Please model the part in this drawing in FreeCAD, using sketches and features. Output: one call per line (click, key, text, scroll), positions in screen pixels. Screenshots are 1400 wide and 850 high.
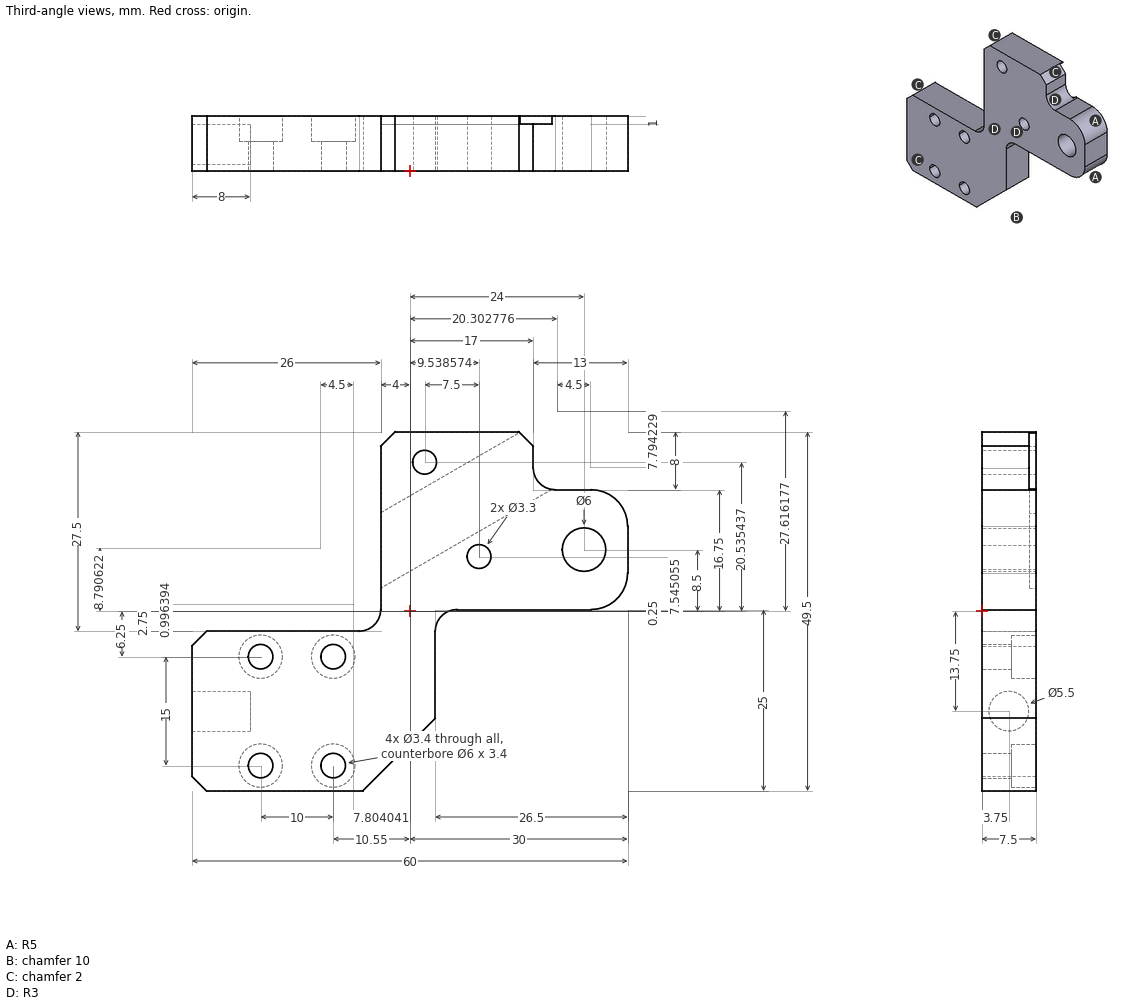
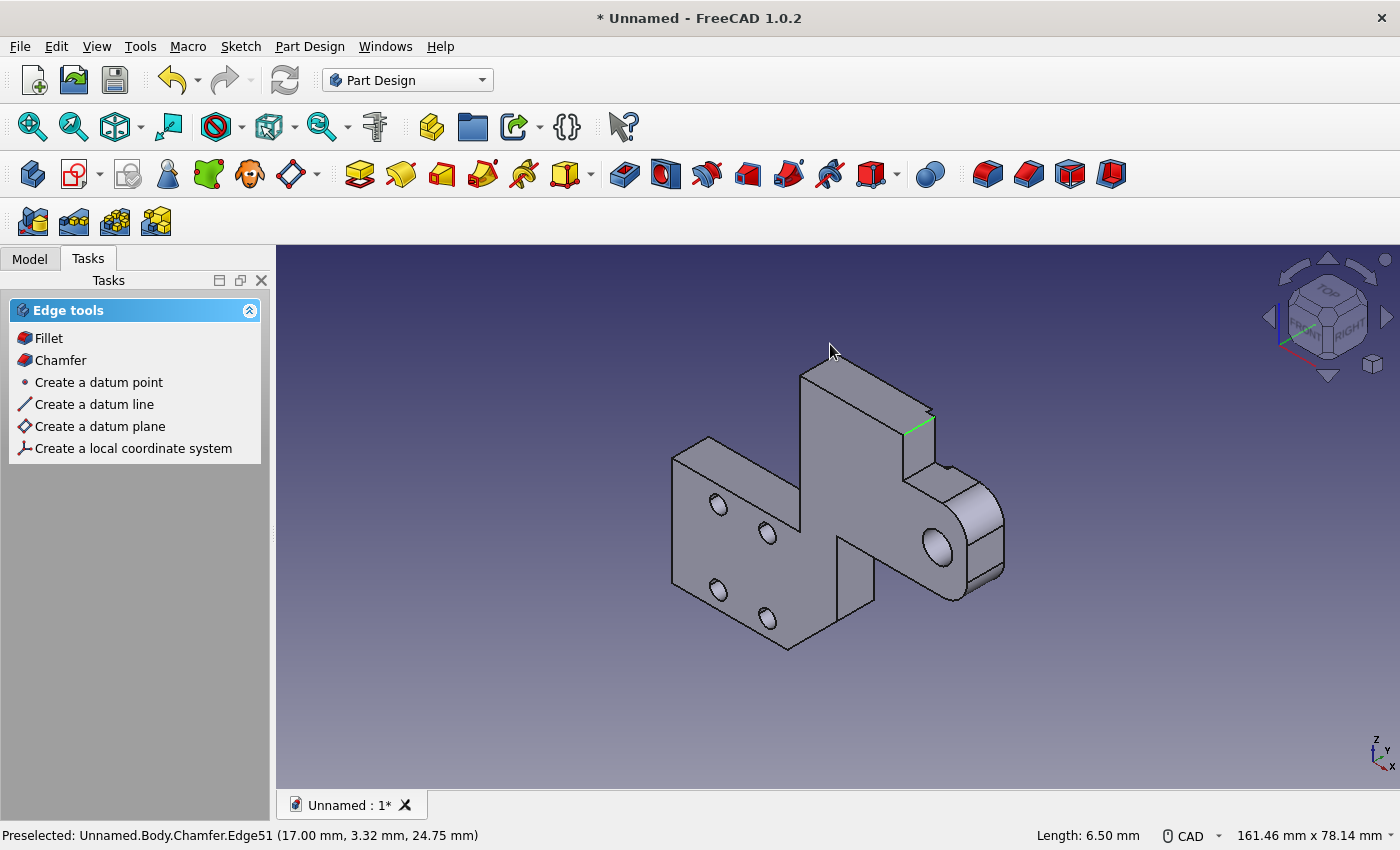
key(2)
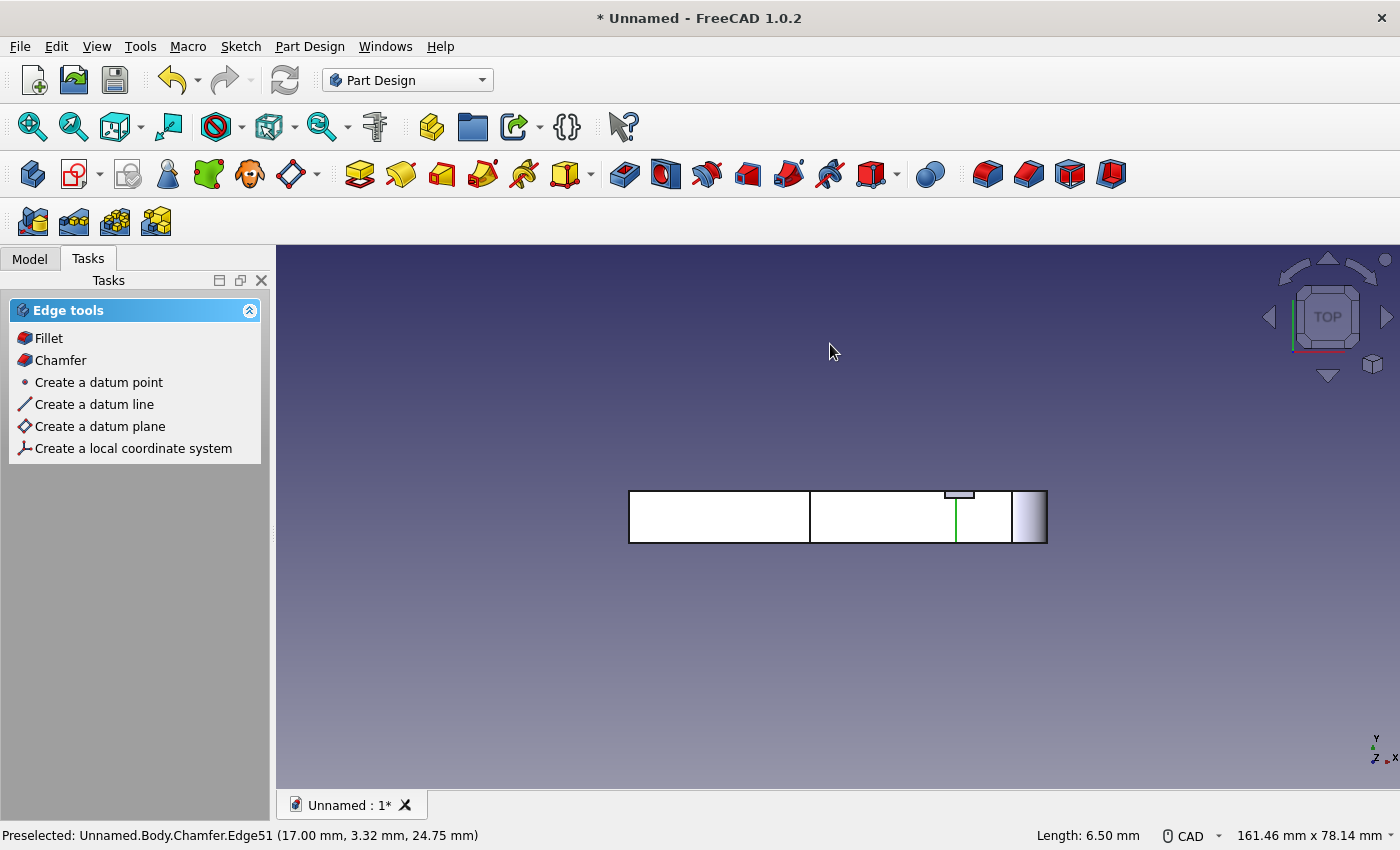
key(v)
key(f)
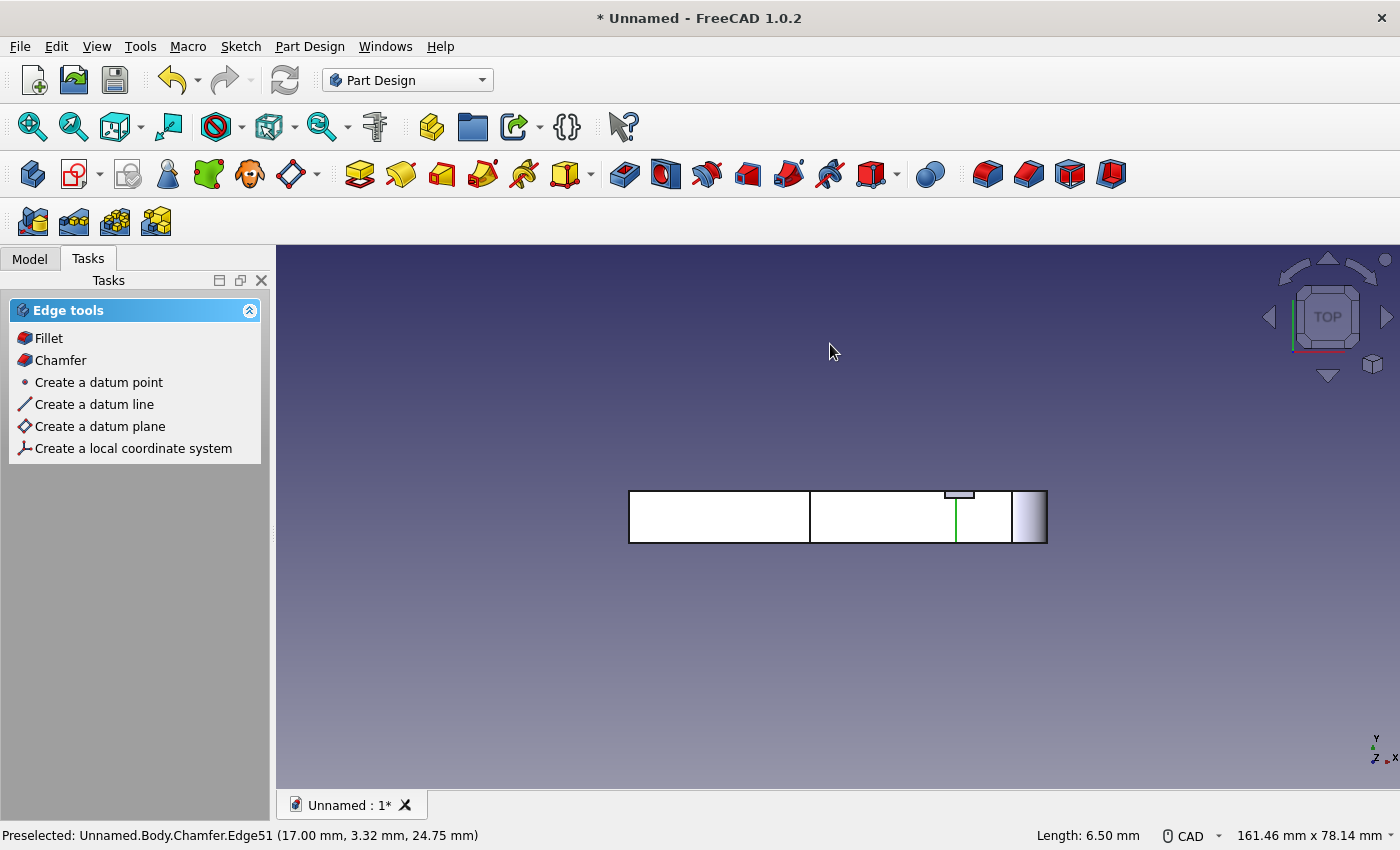
click(810, 516, ctrl)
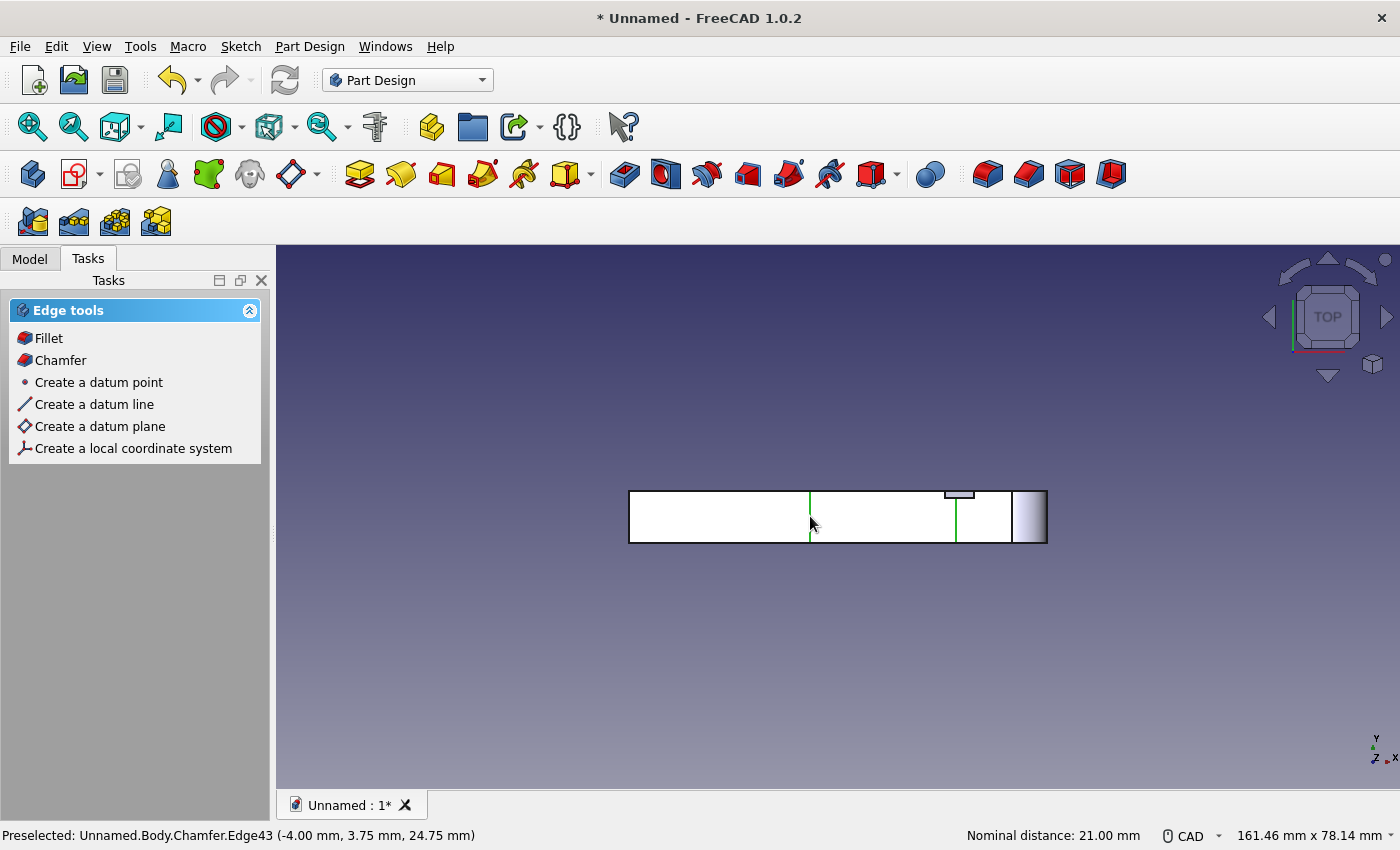
click(629, 516, ctrl)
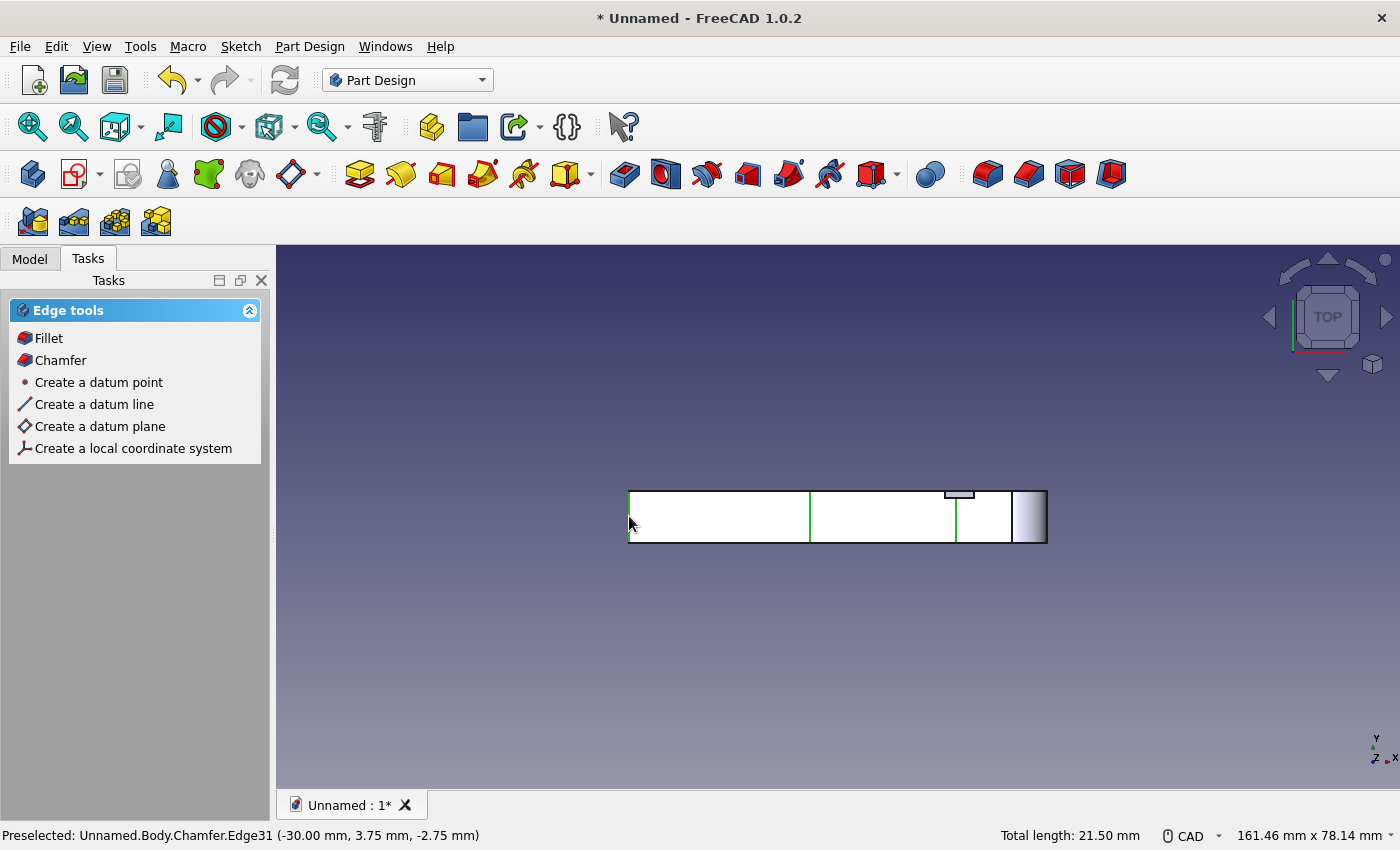
key(1)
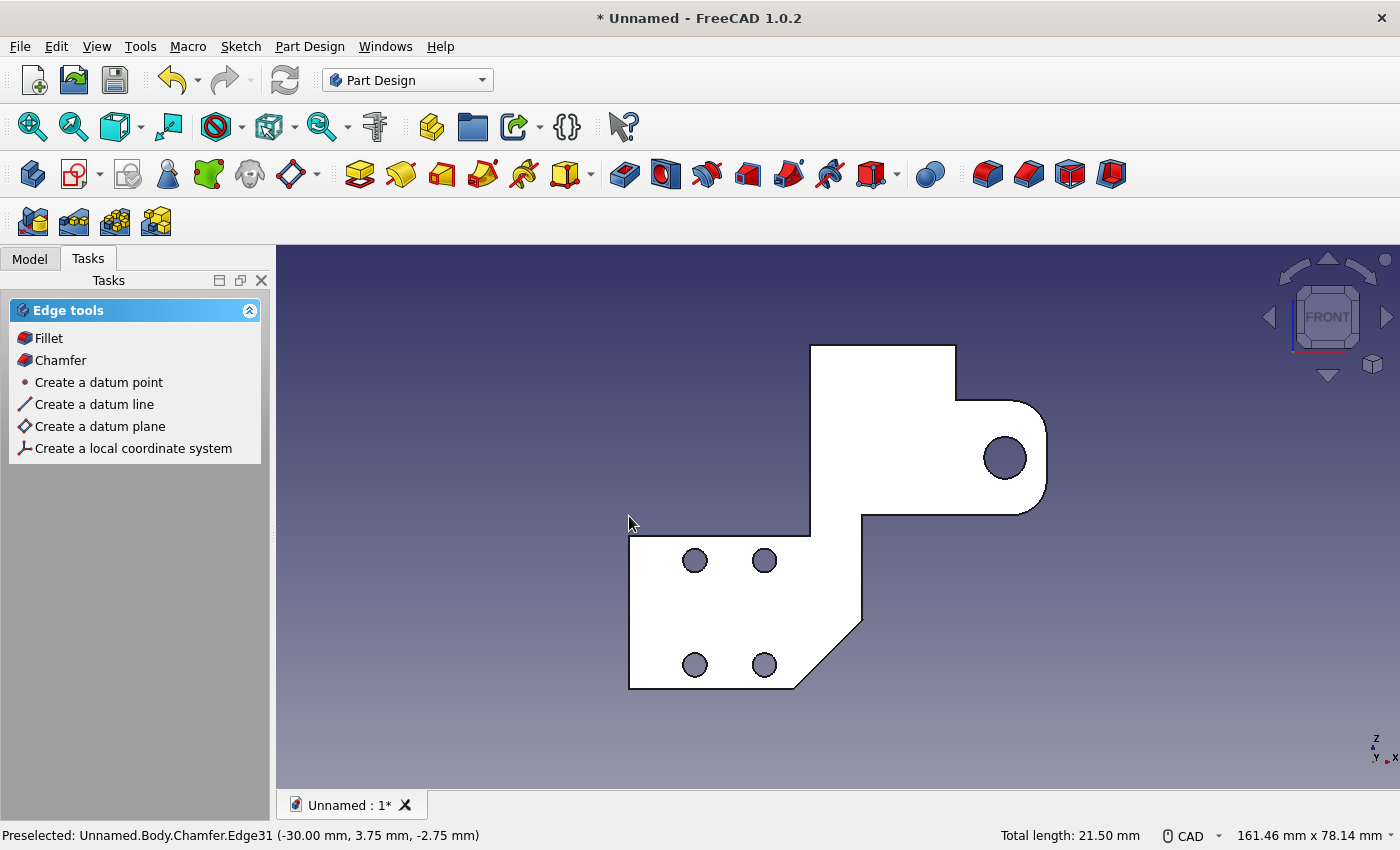
key(3)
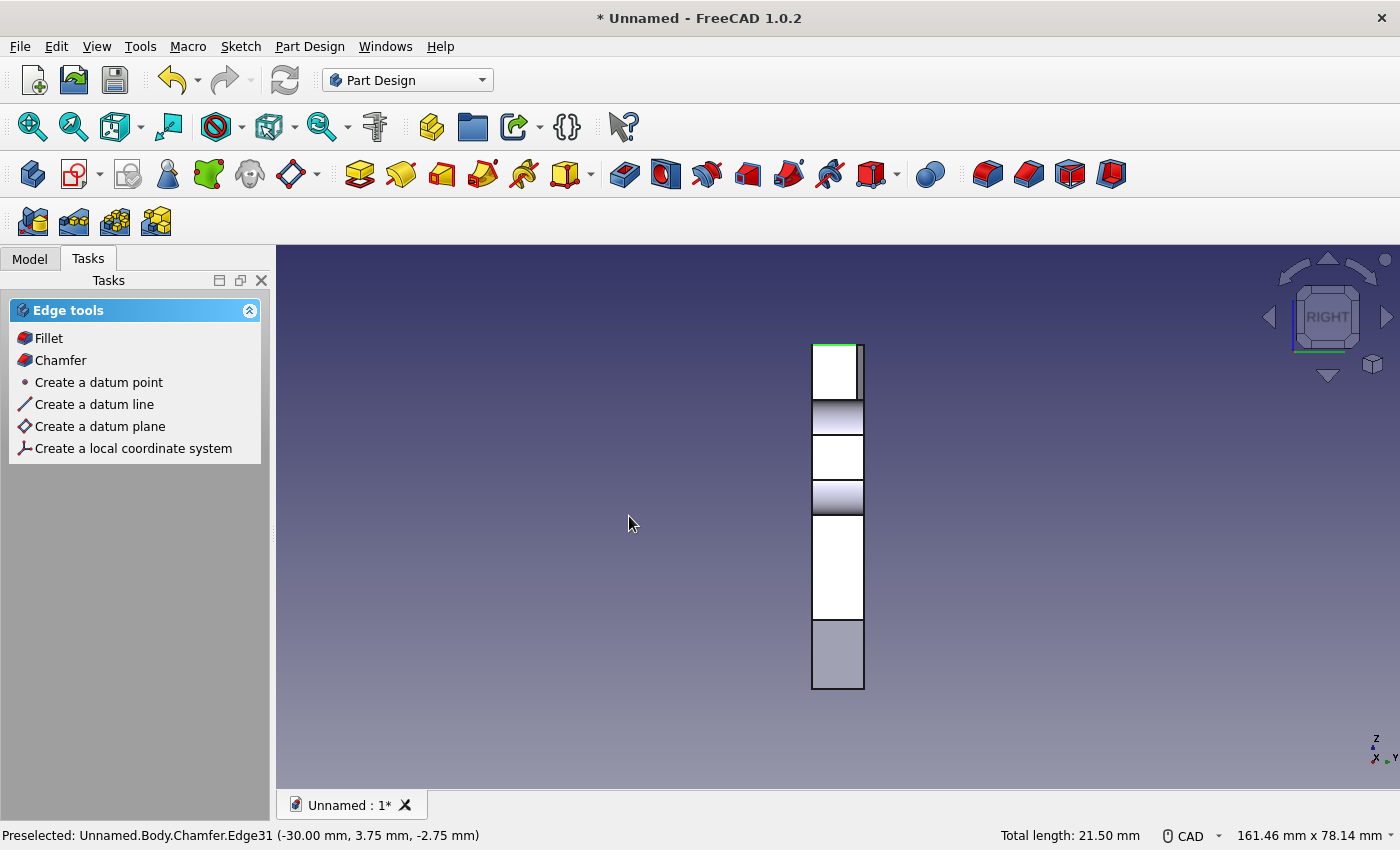
key(5)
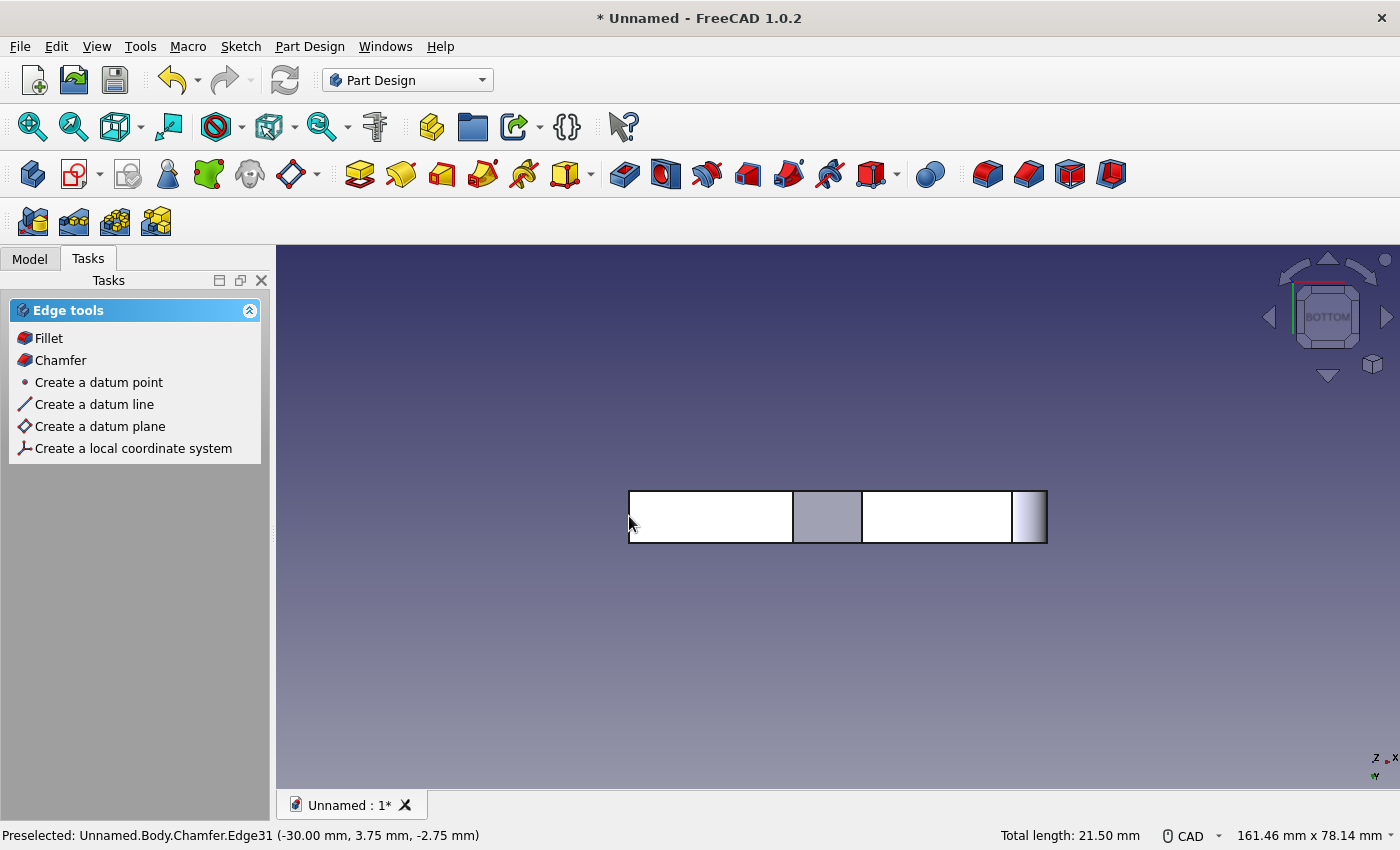
key(v)
key(f)